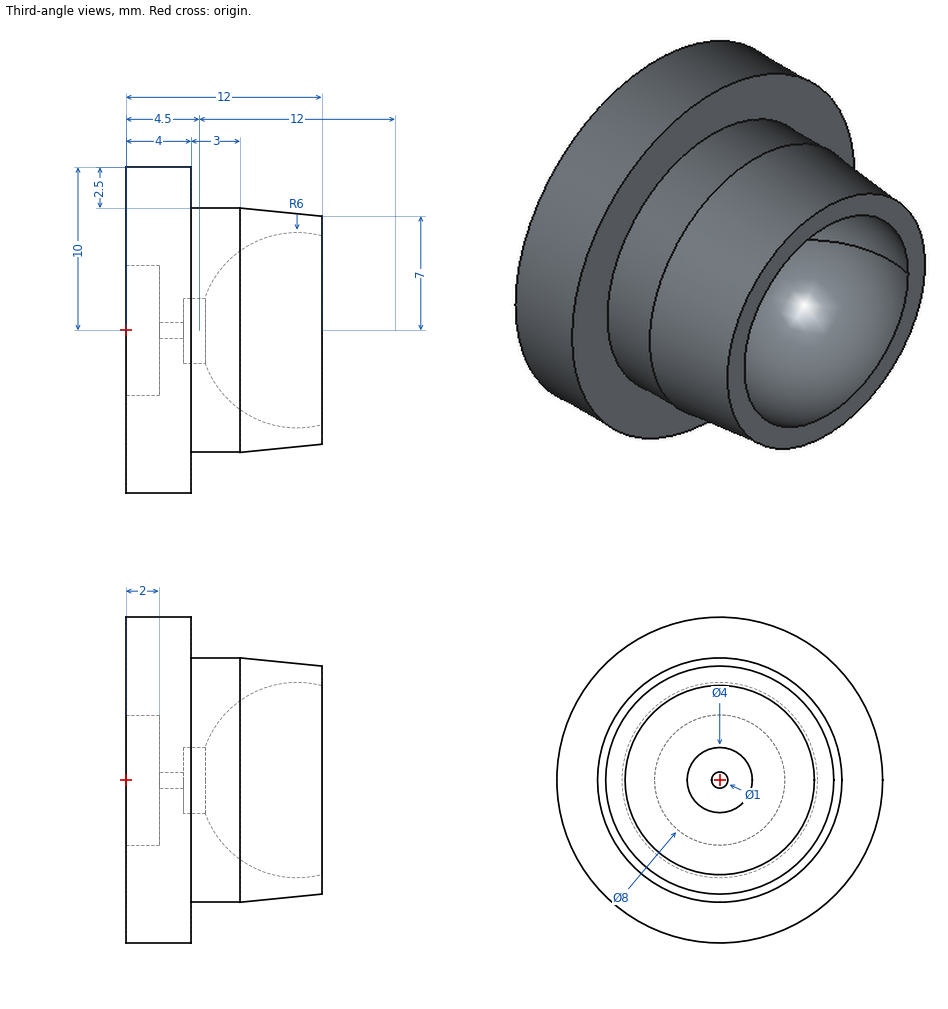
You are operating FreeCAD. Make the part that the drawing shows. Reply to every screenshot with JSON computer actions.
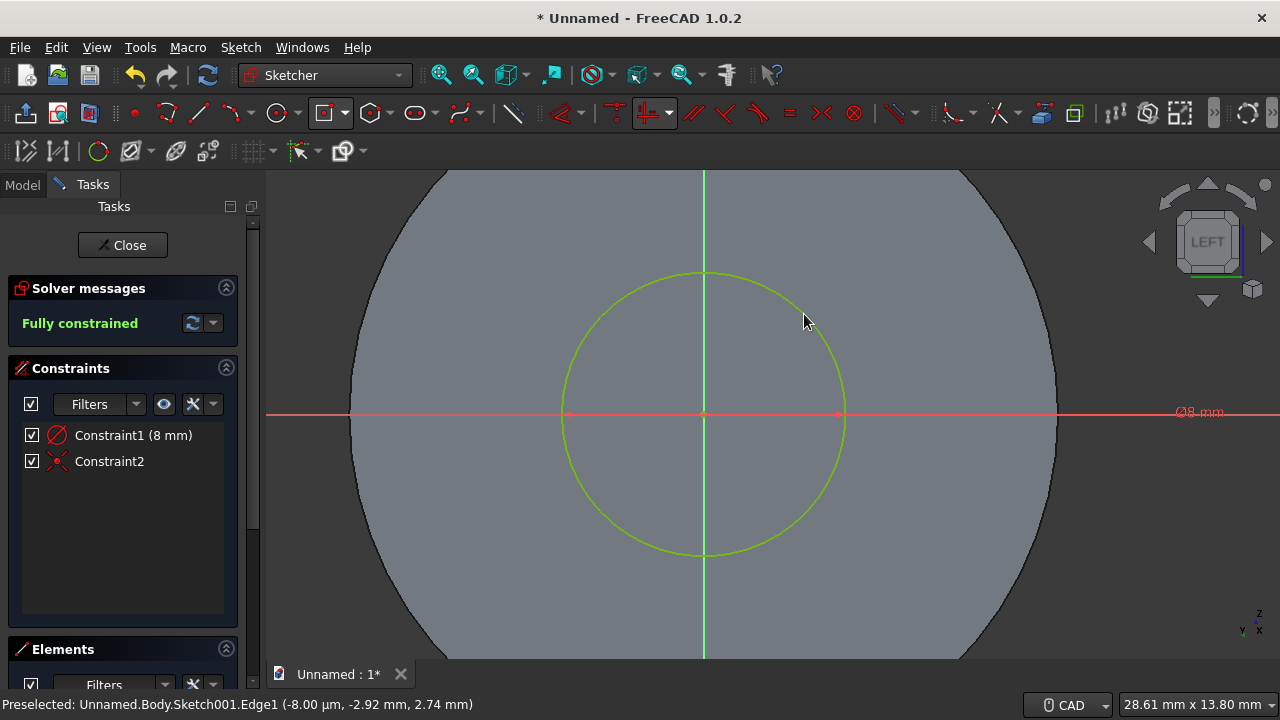
{"action": "left_click", "coordinate": [123, 245]}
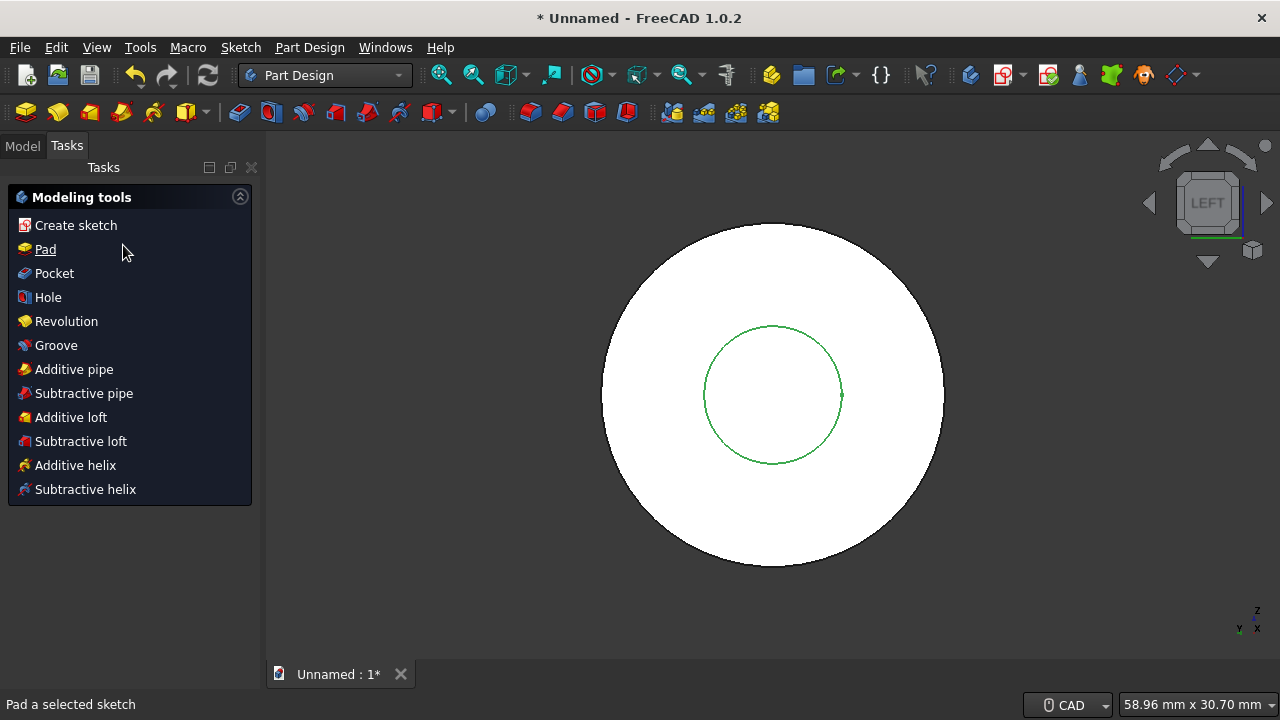
{"action": "left_click", "coordinate": [240, 112]}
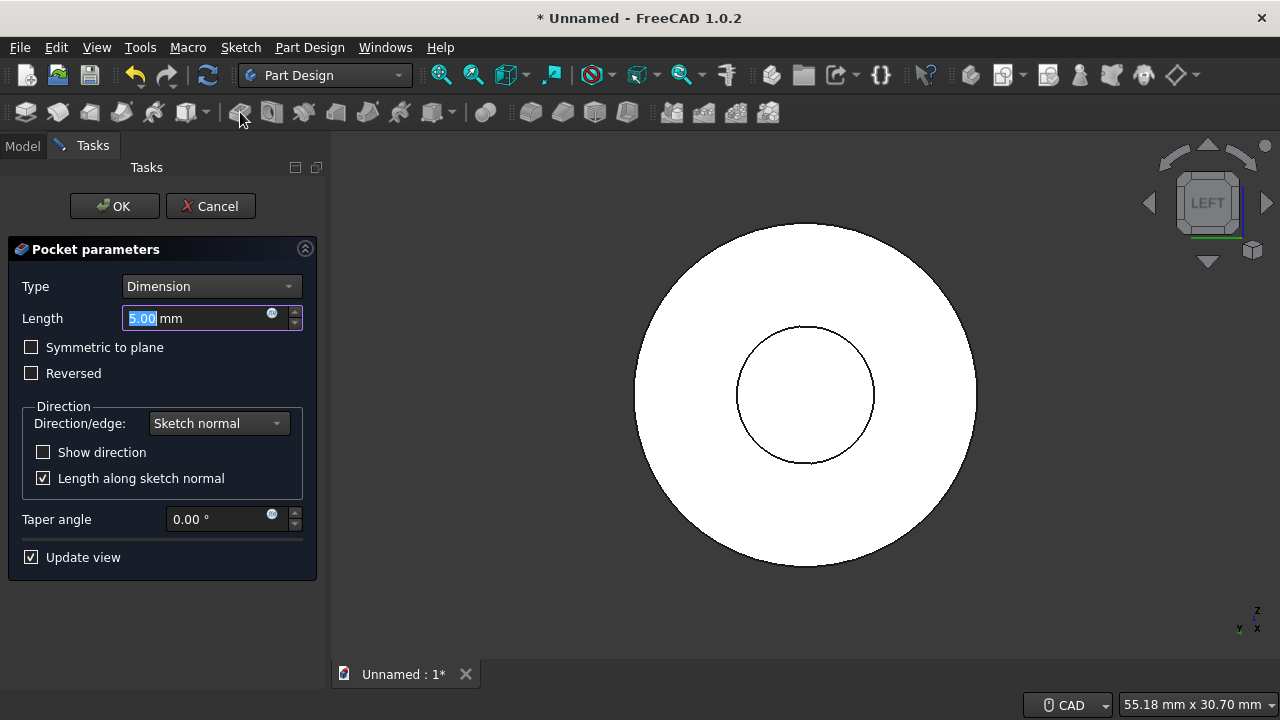
{"action": "type", "text": "2"}
{"action": "key", "text": "Tab"}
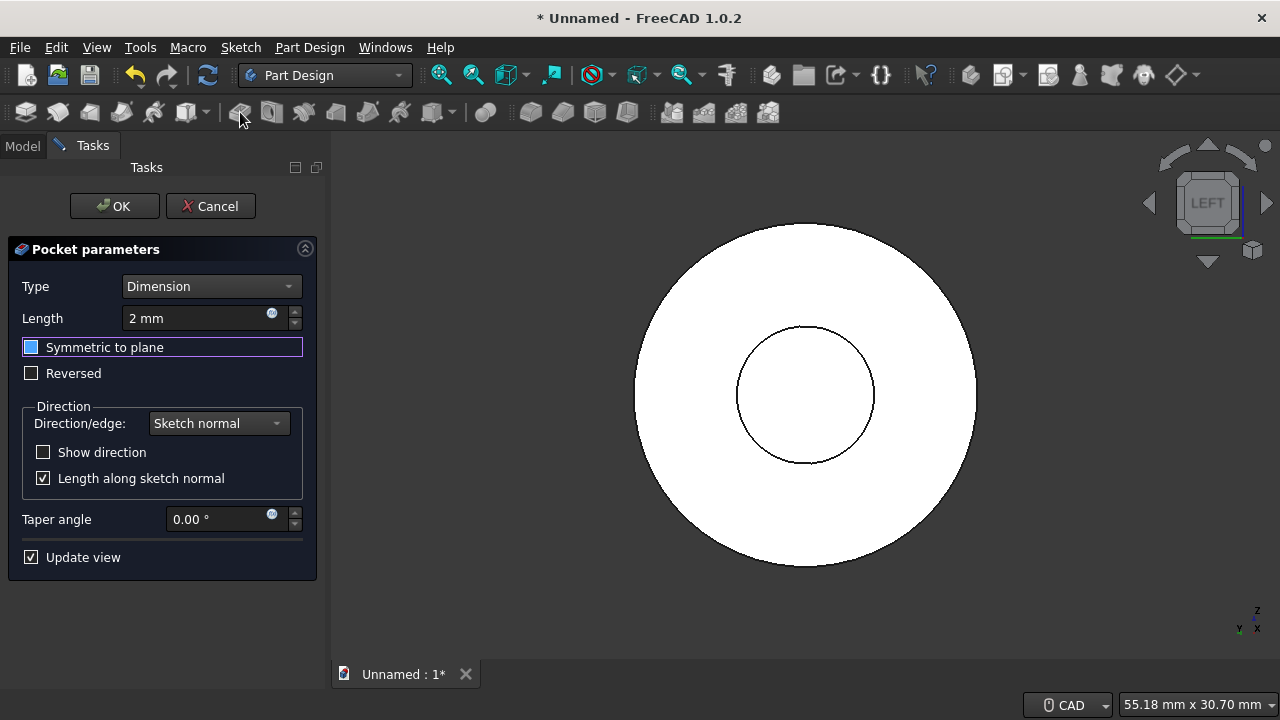
{"action": "left_click", "coordinate": [115, 206]}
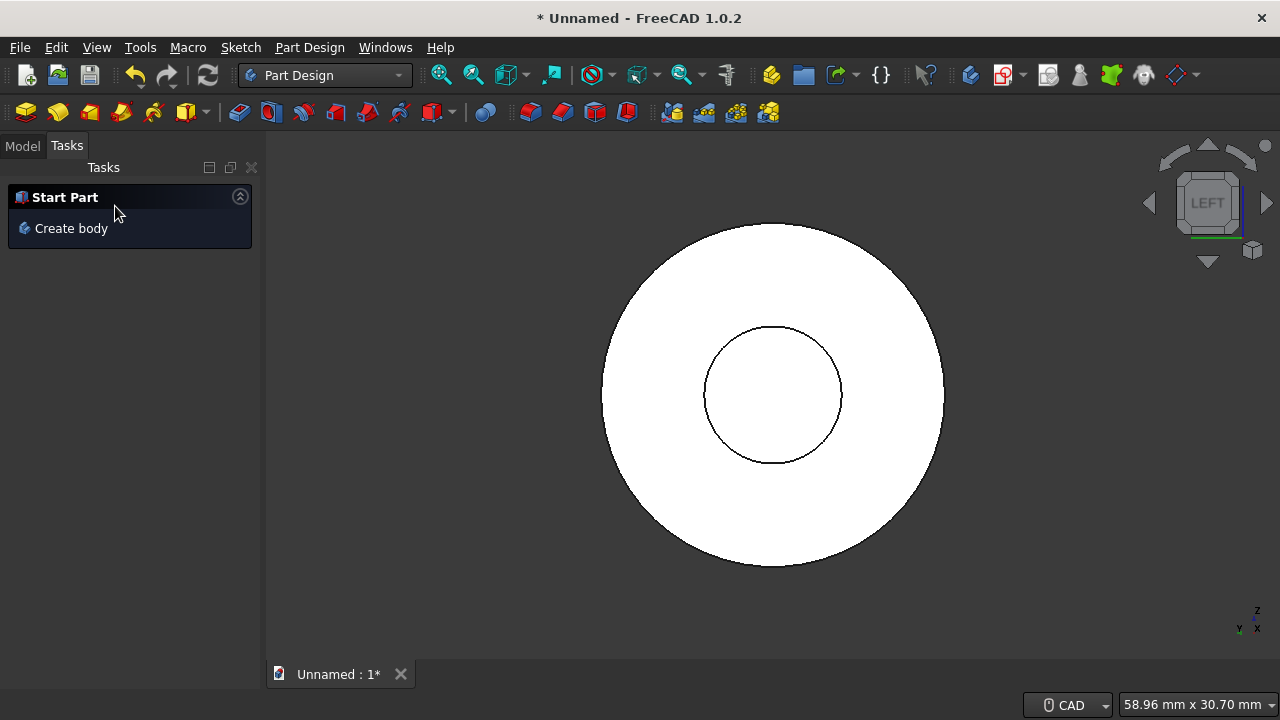
{"action": "left_click", "coordinate": [773, 394]}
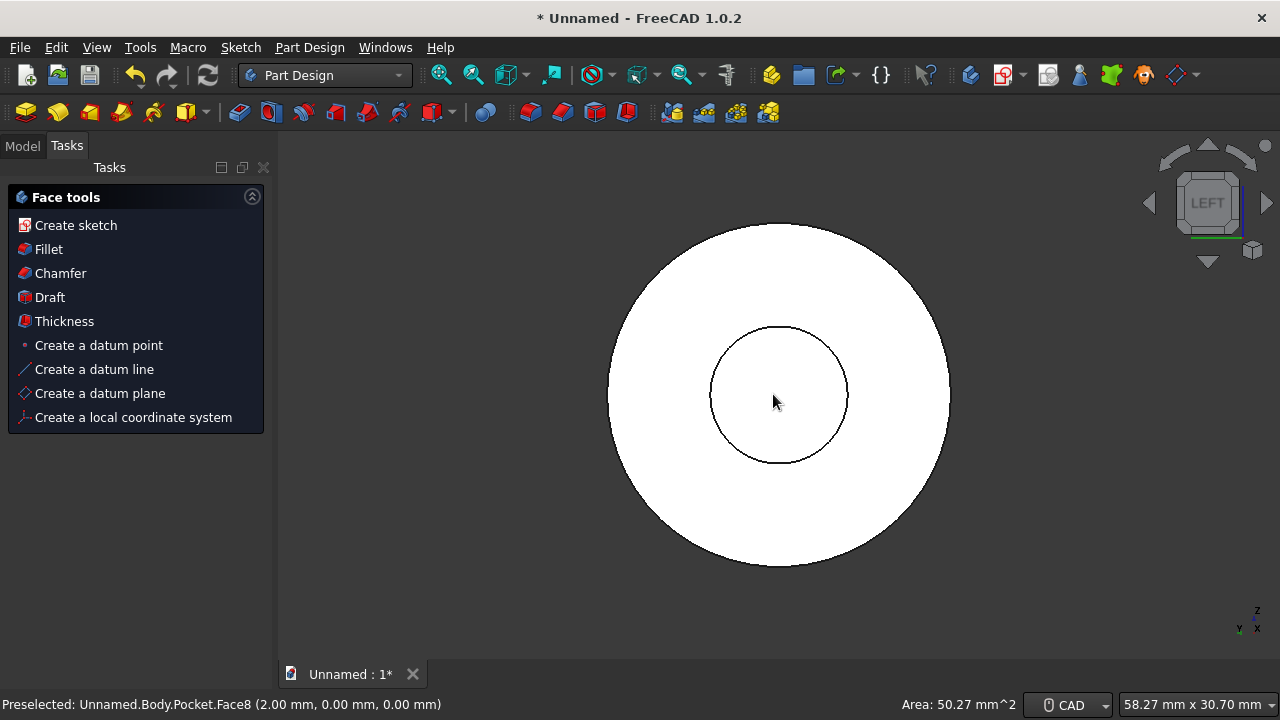
{"action": "left_click", "coordinate": [1004, 76]}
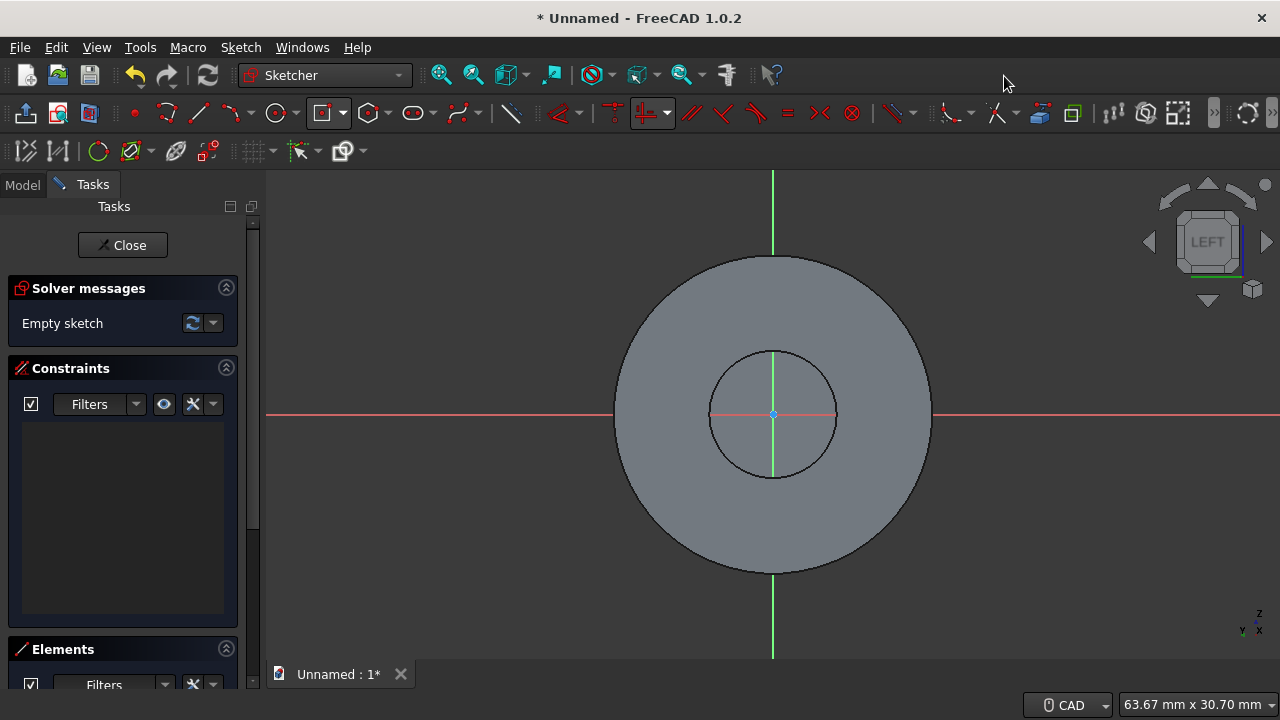
{"action": "left_click", "coordinate": [90, 114]}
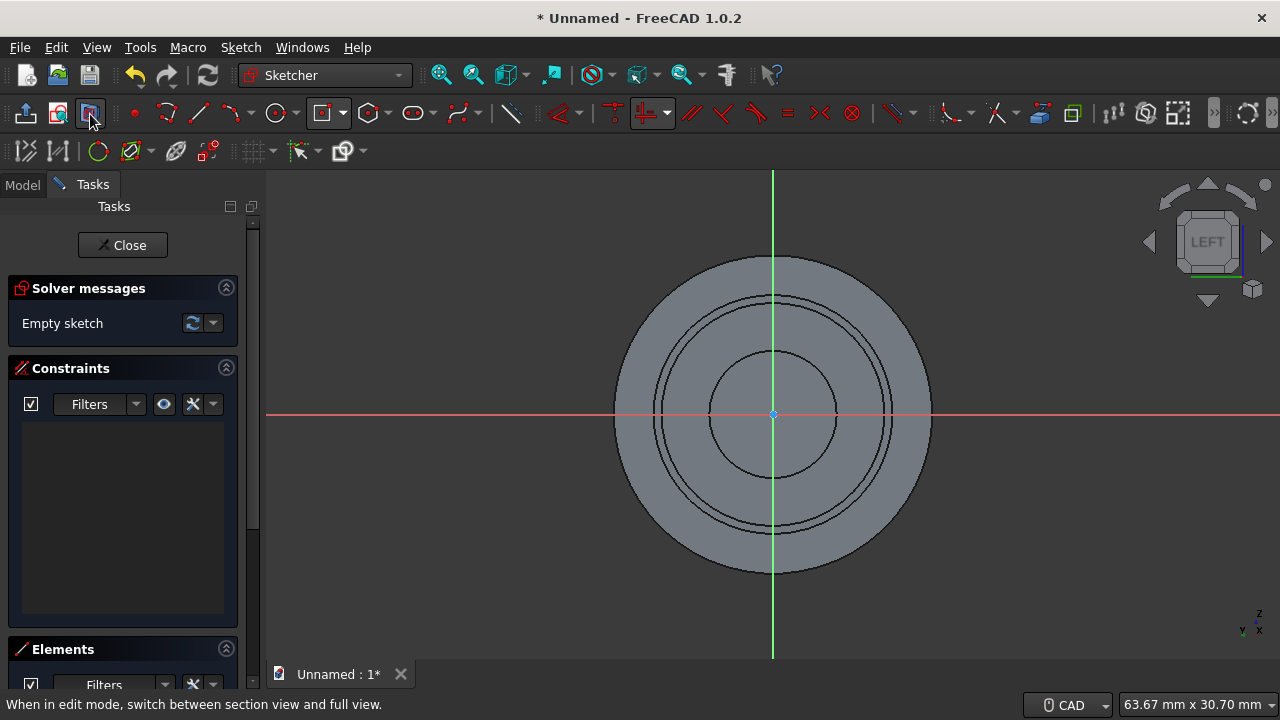
{"action": "scroll", "coordinate": [777, 415], "scroll_direction": "up", "scroll_amount": 15}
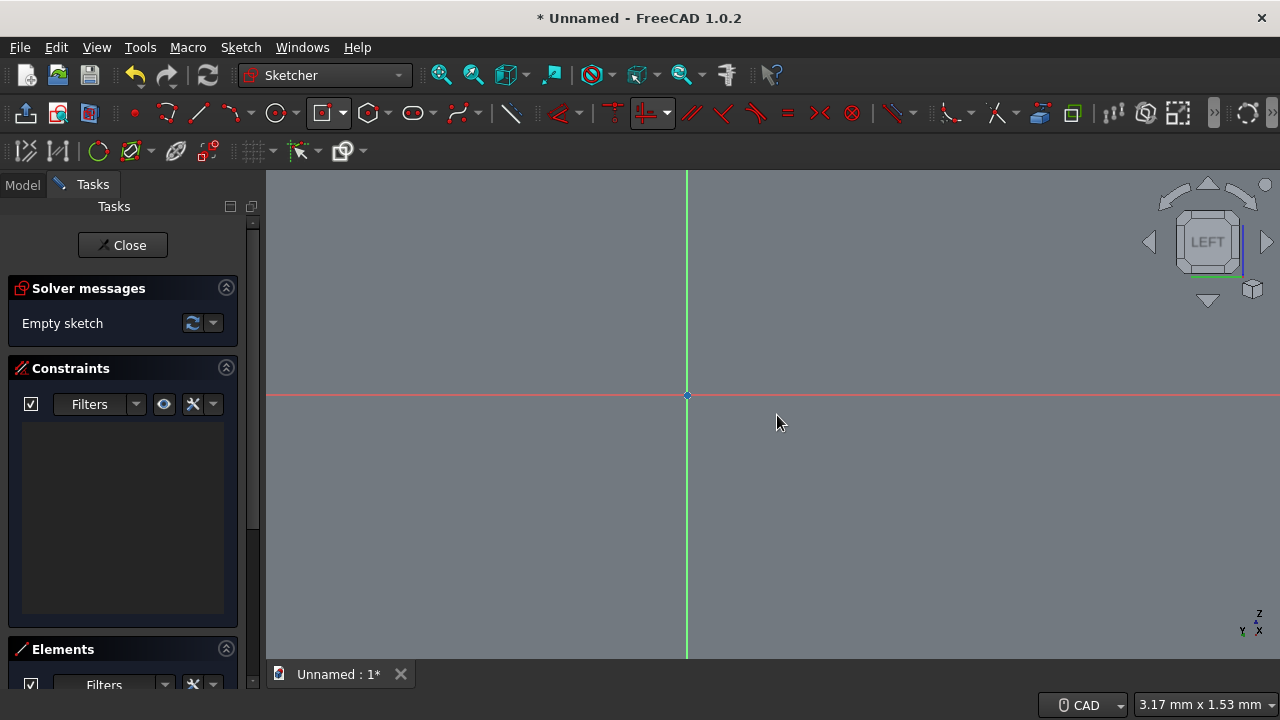
{"action": "left_click", "coordinate": [276, 114]}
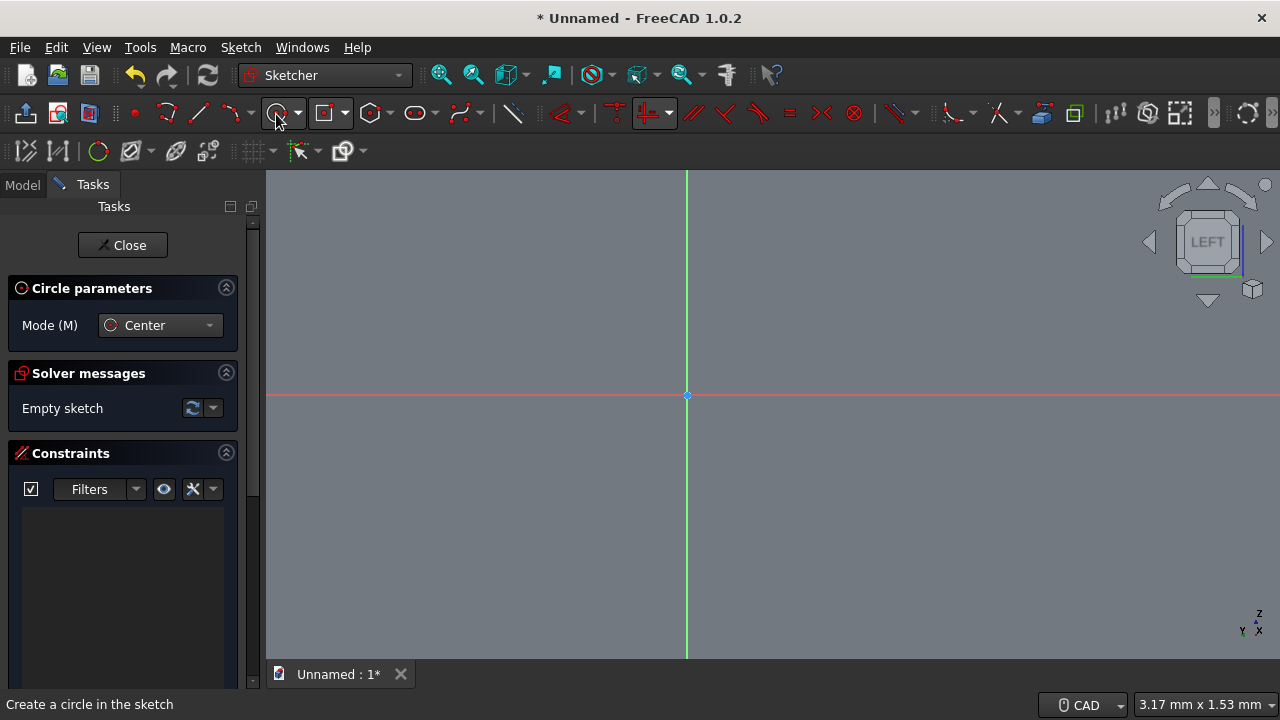
{"action": "left_click", "coordinate": [687, 395]}
{"action": "mouse_move", "coordinate": [800, 282]}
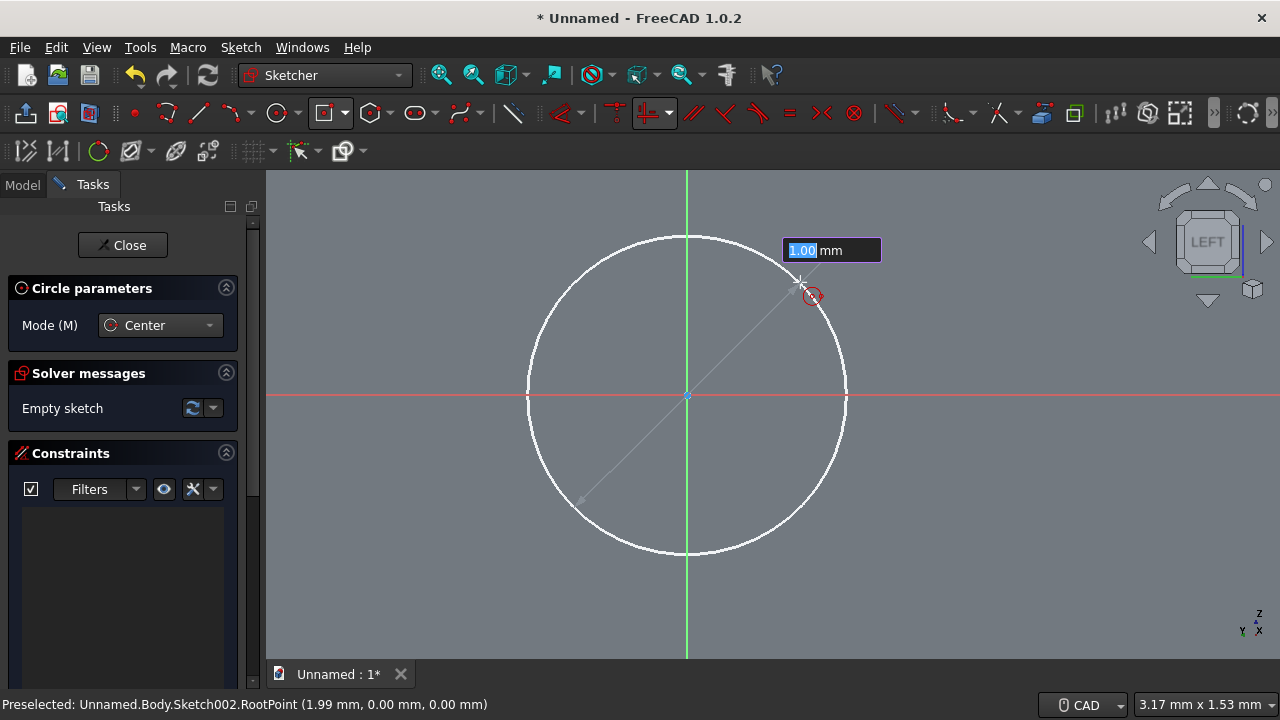
{"action": "type", "text": "1"}
{"action": "key", "text": "Return"}
{"action": "key", "text": "Escape"}